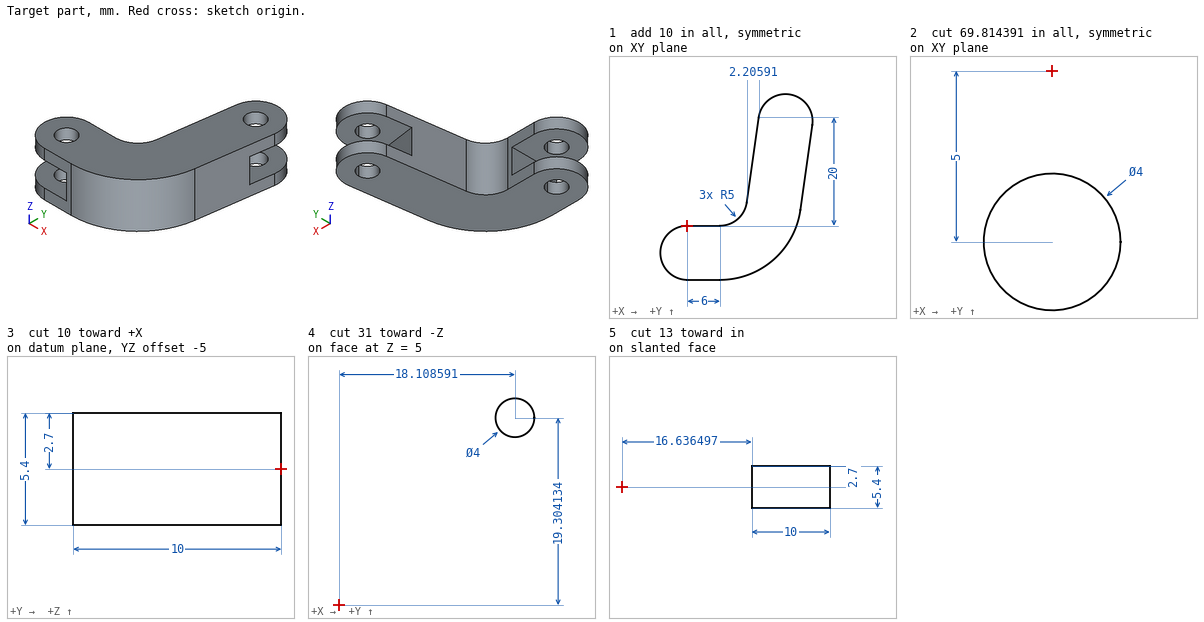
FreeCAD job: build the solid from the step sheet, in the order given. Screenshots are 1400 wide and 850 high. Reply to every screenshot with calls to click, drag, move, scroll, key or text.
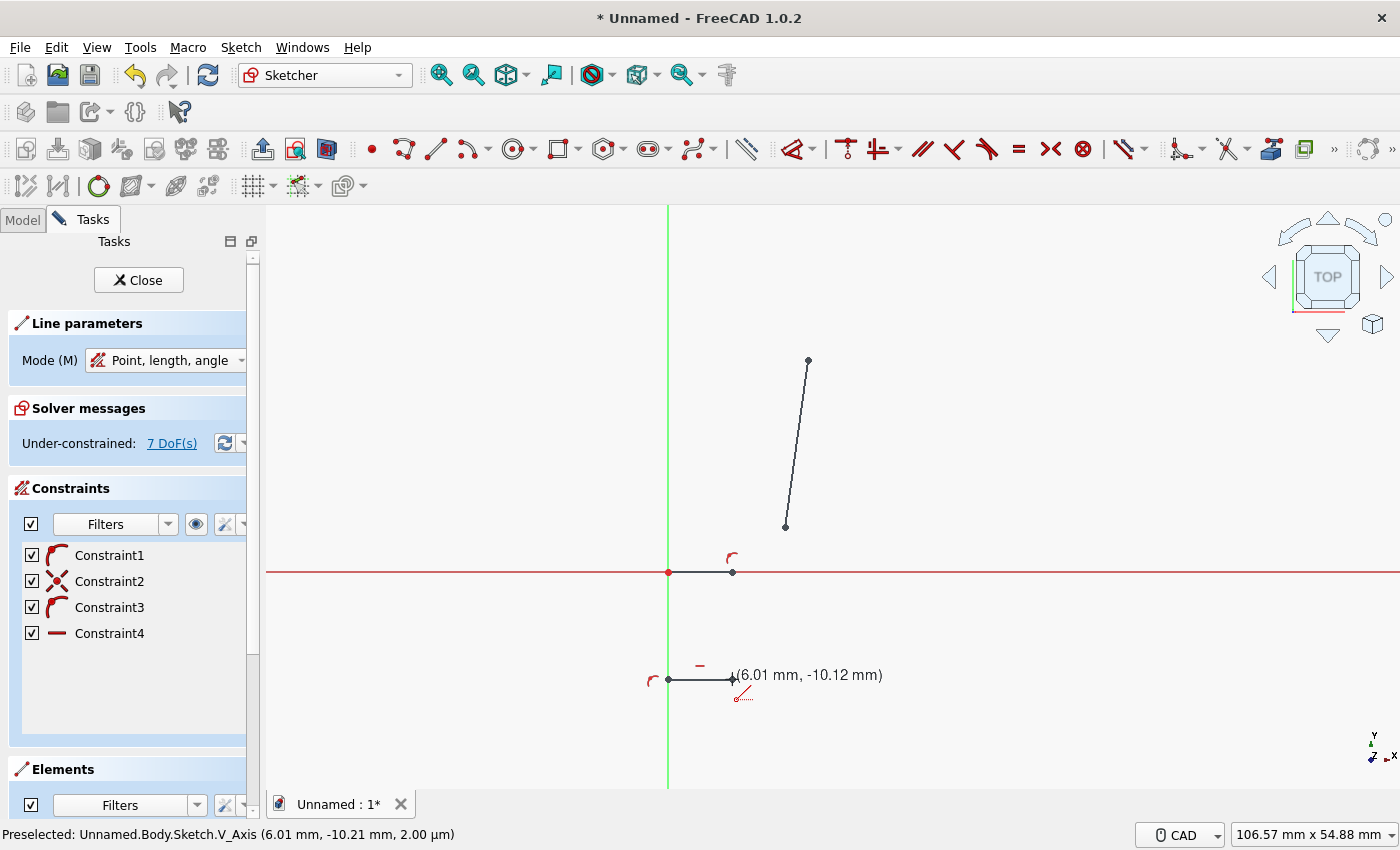
click(890, 541)
click(913, 374)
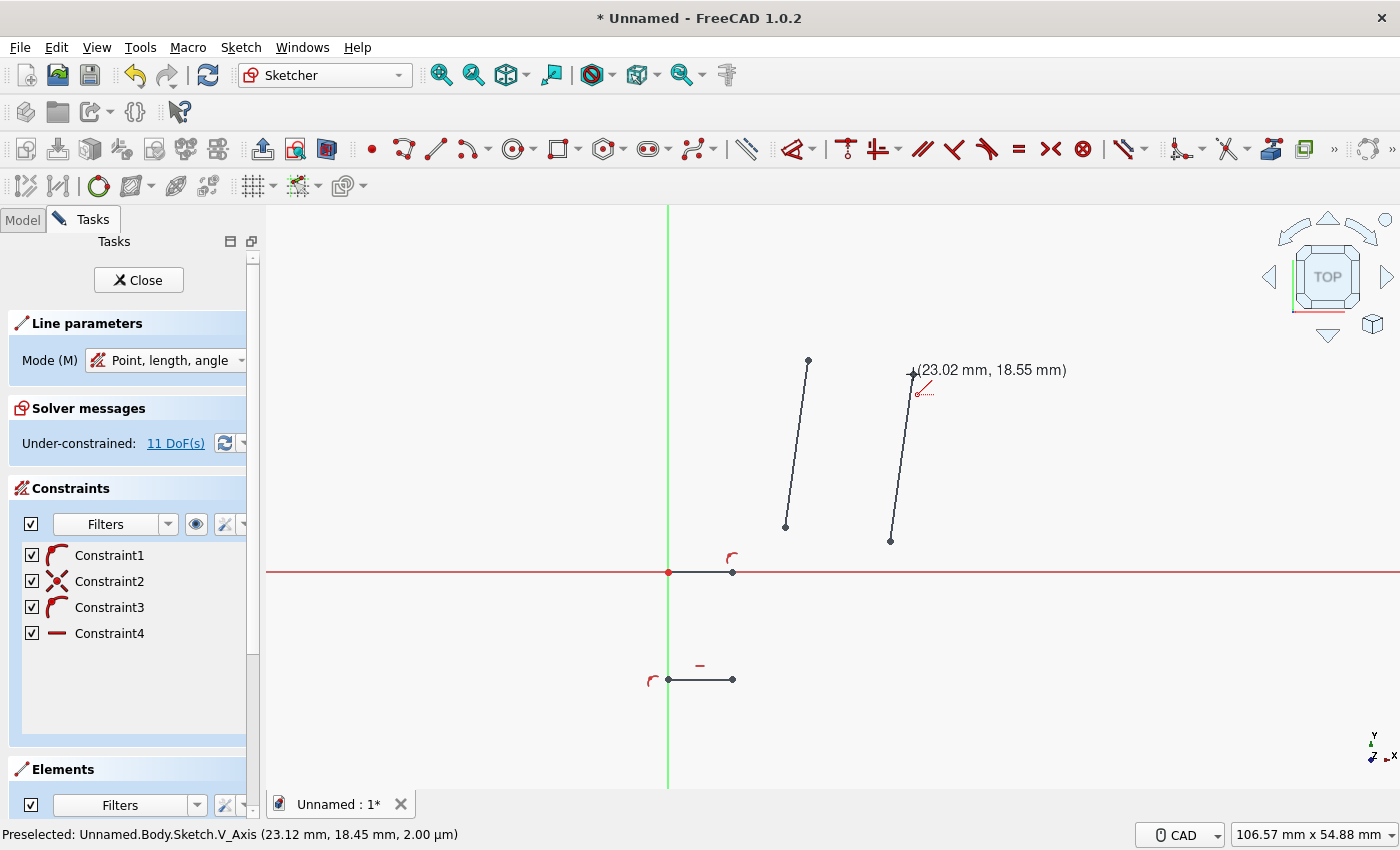
click(490, 150)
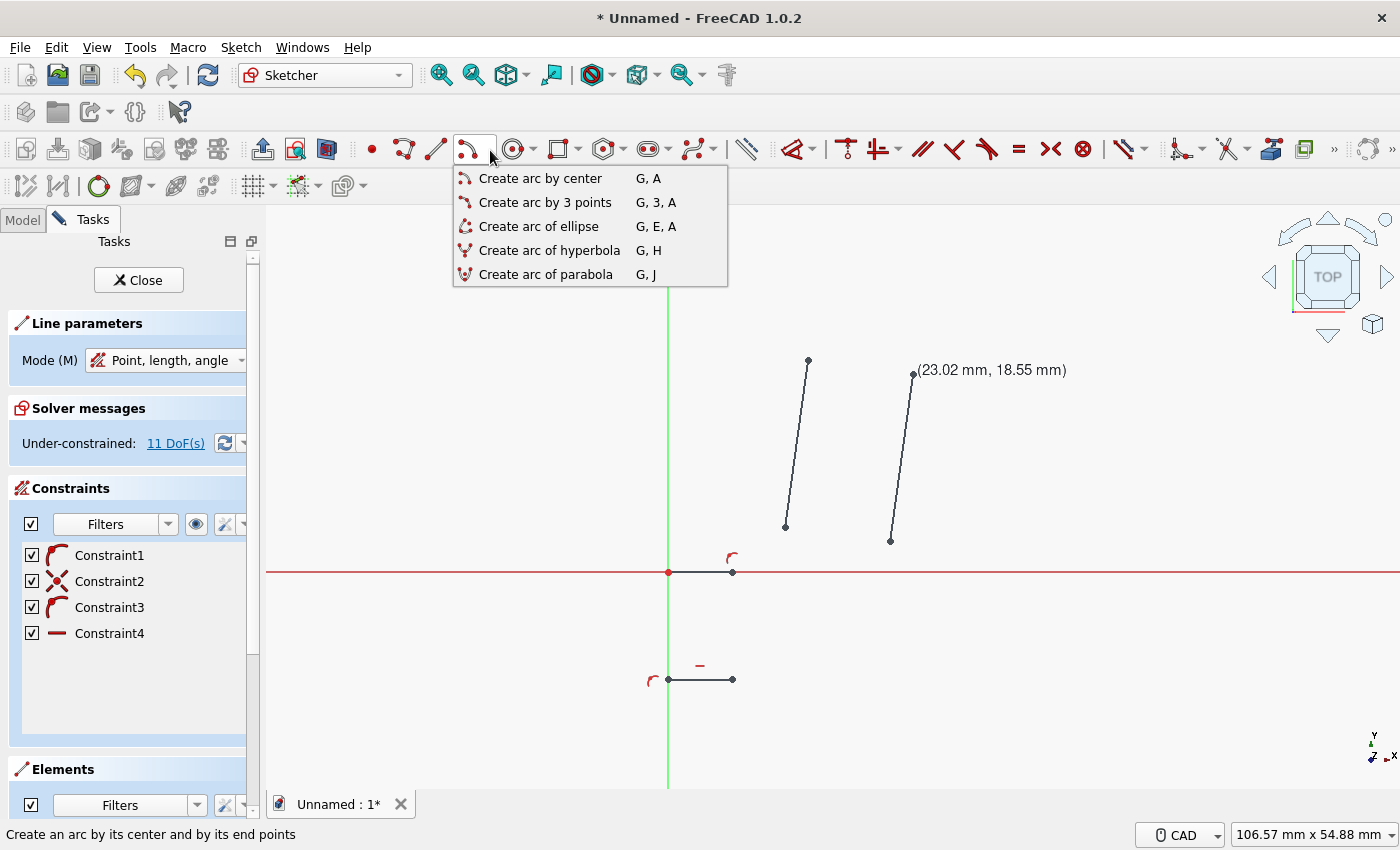
click(590, 202)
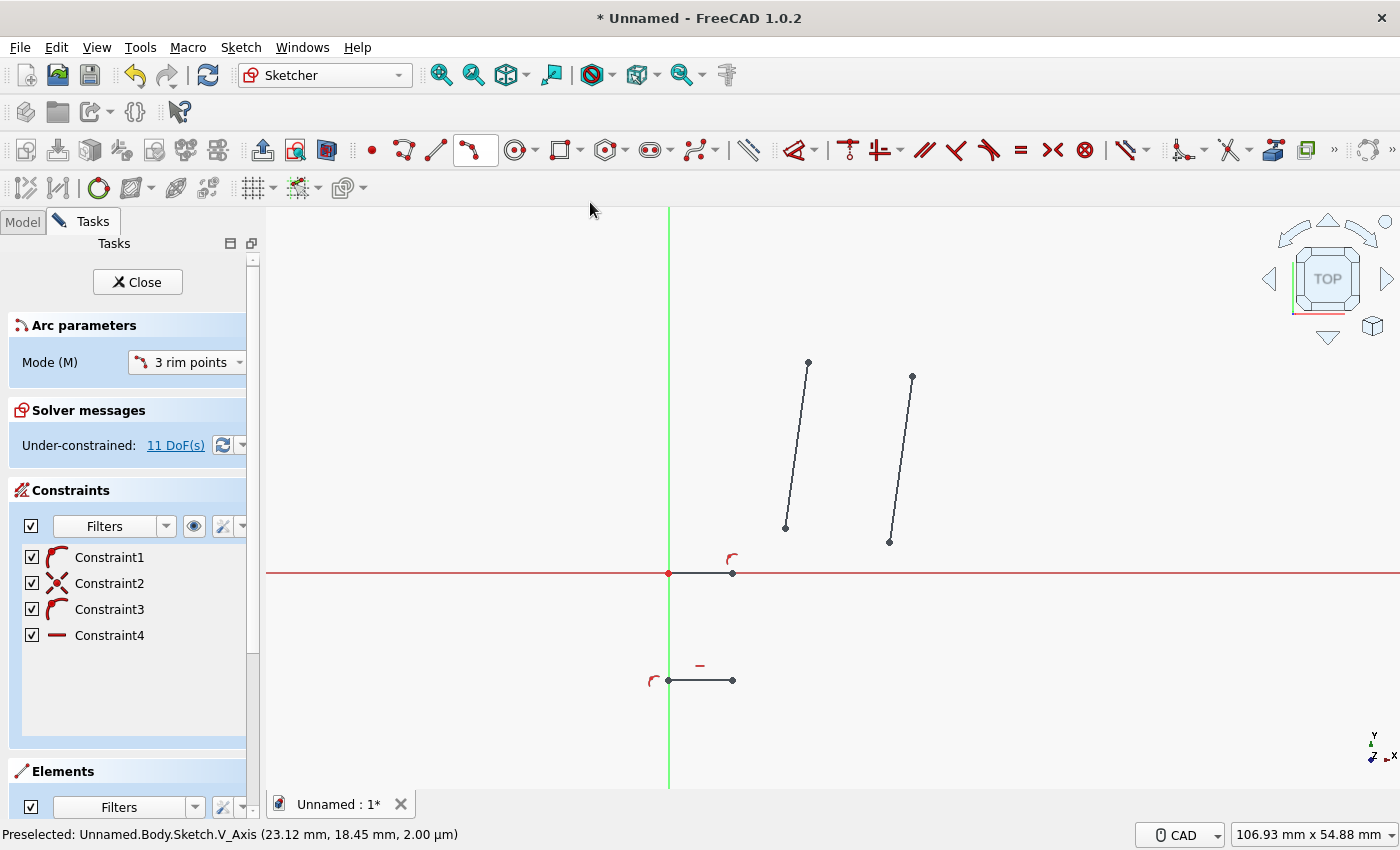
click(785, 529)
click(732, 573)
click(767, 560)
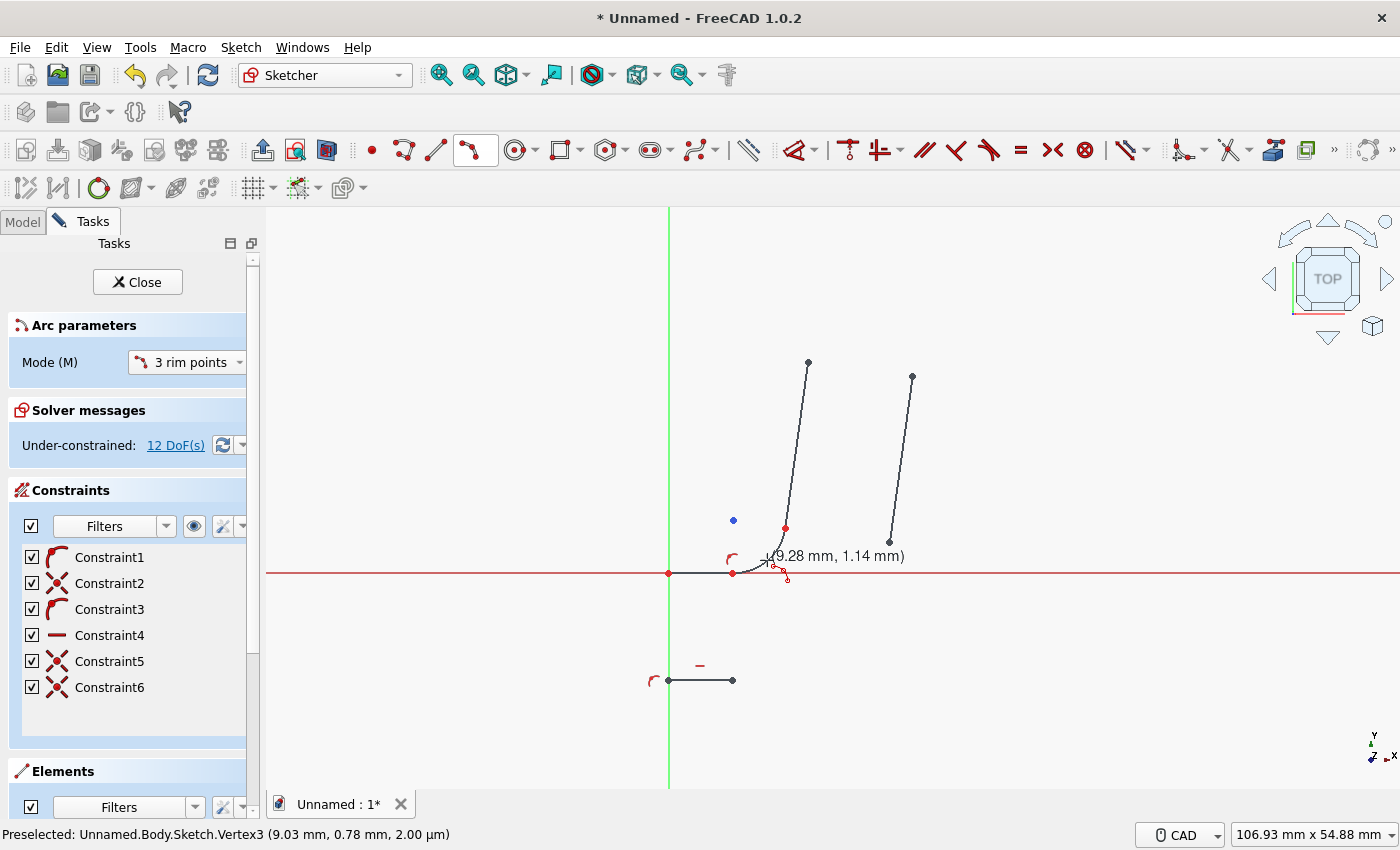
click(669, 573)
click(669, 680)
click(616, 626)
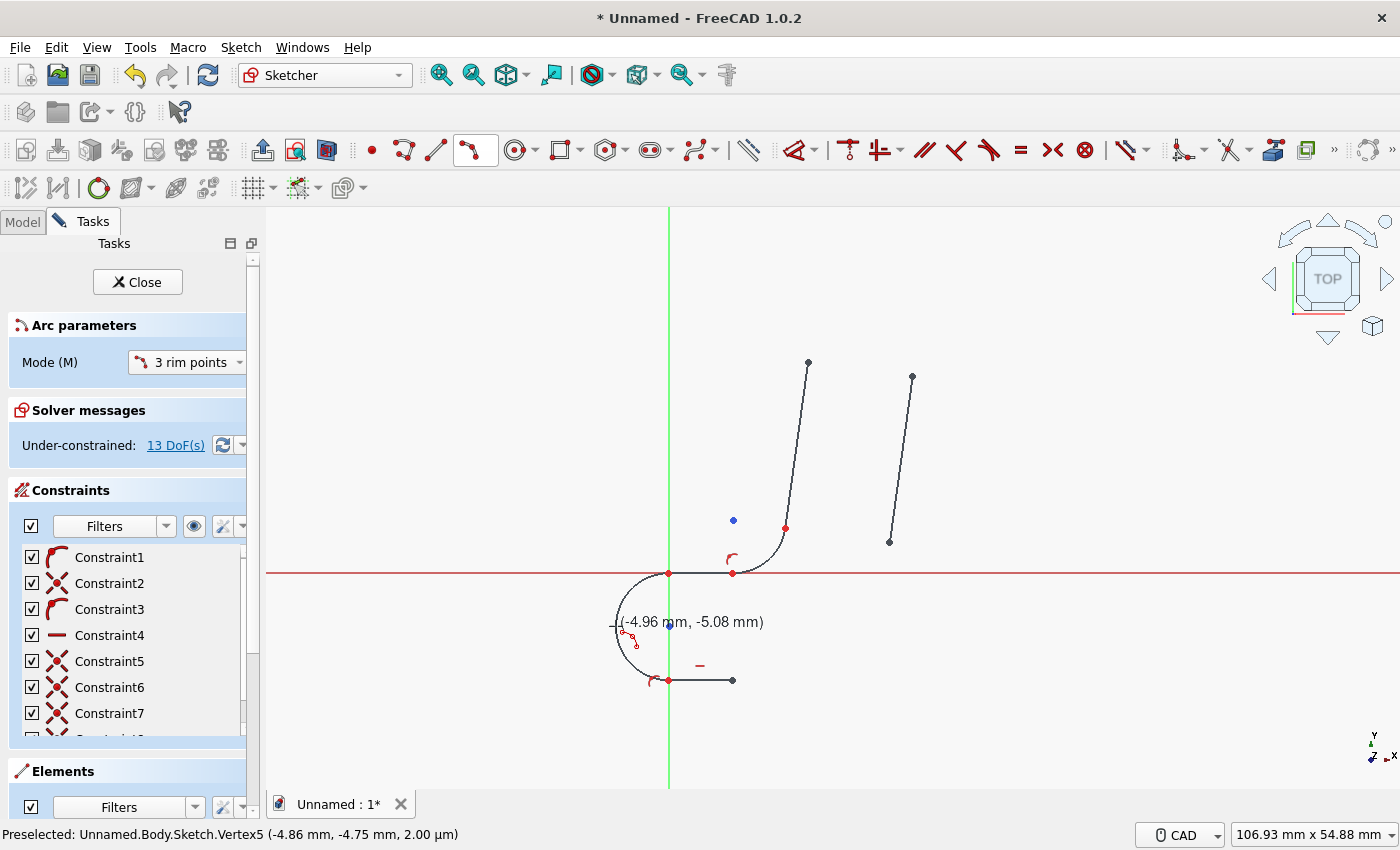
click(732, 680)
click(890, 543)
click(837, 640)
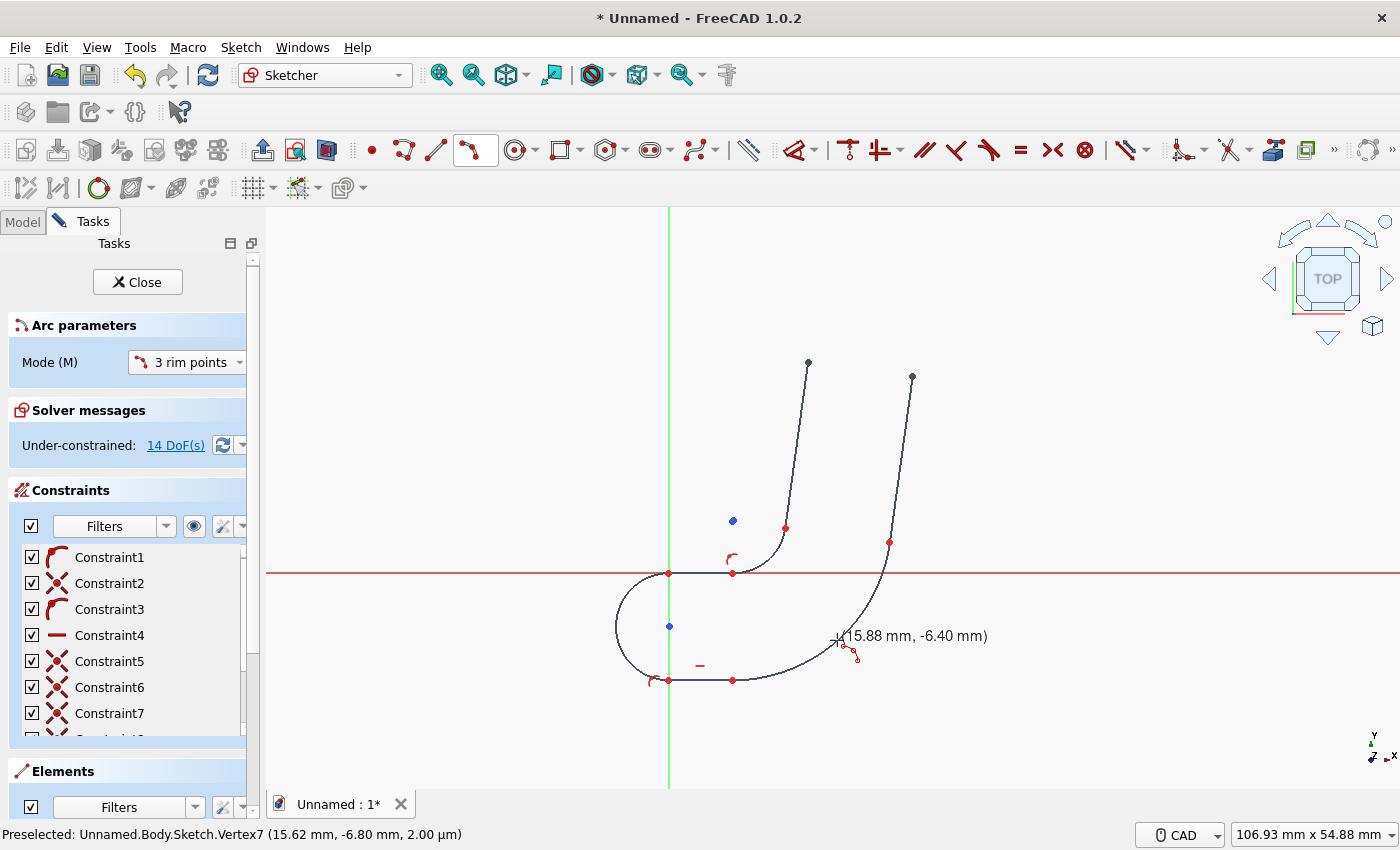
click(913, 376)
click(808, 362)
click(868, 316)
key(Escape)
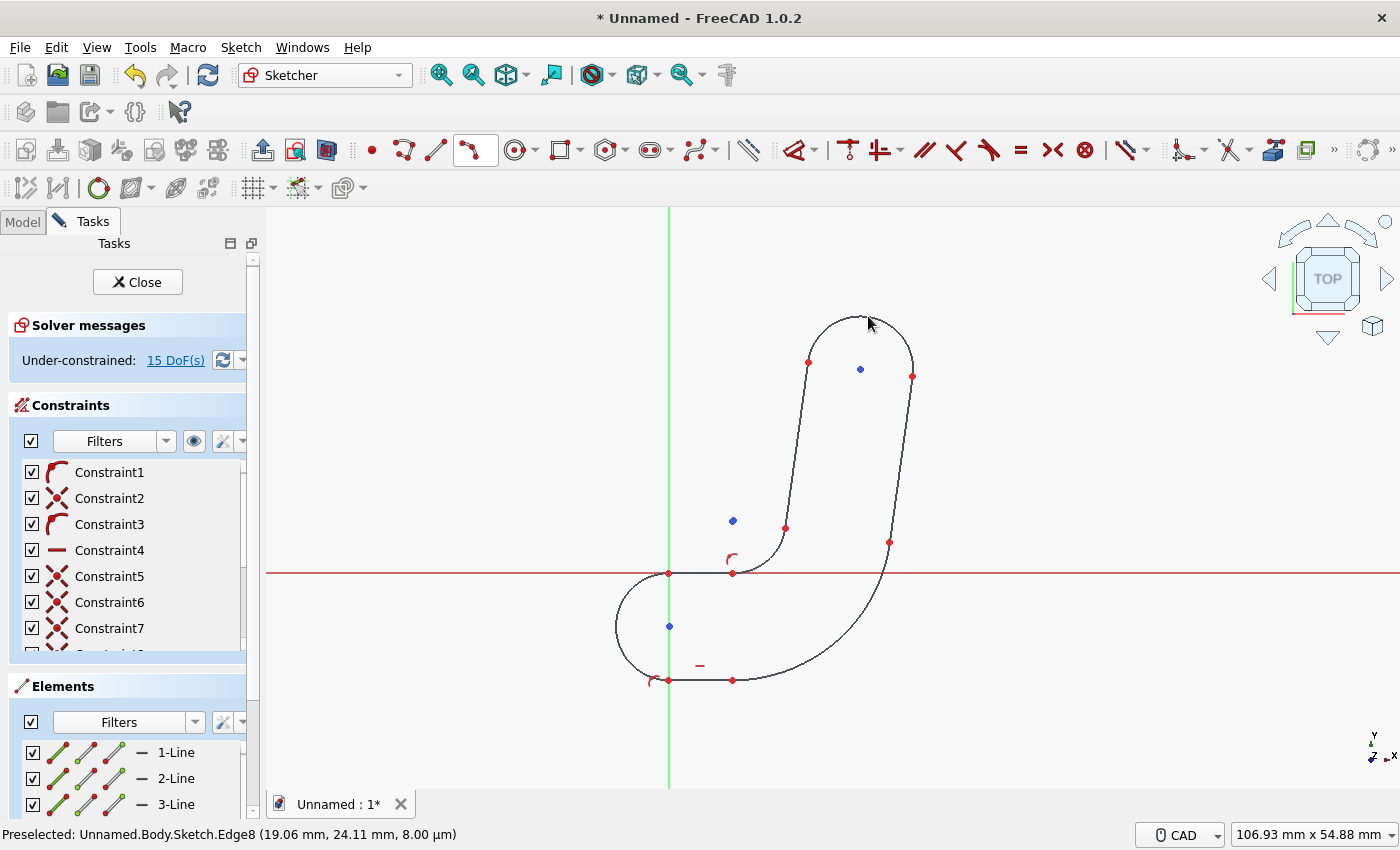
click(801, 412)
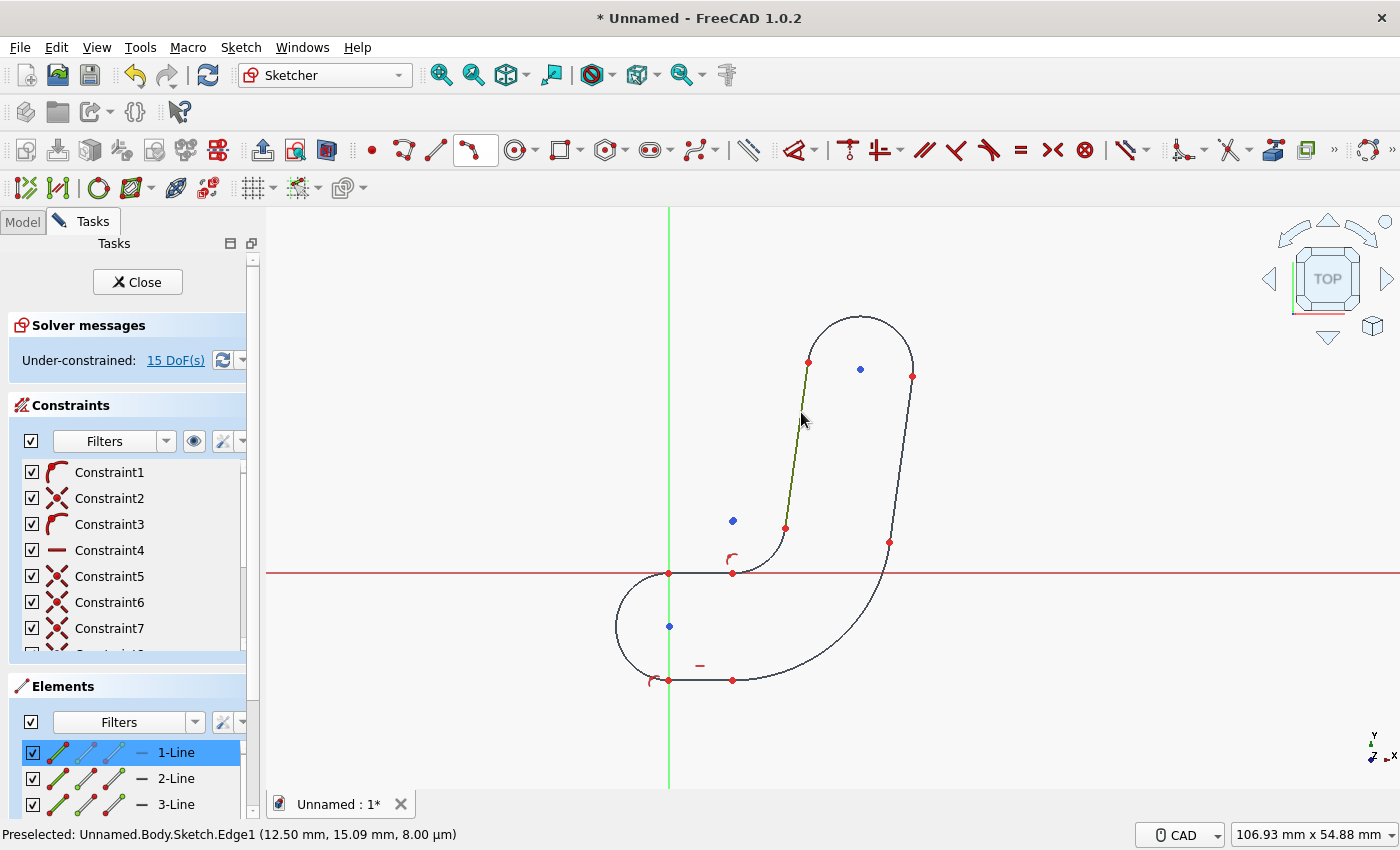
click(777, 550)